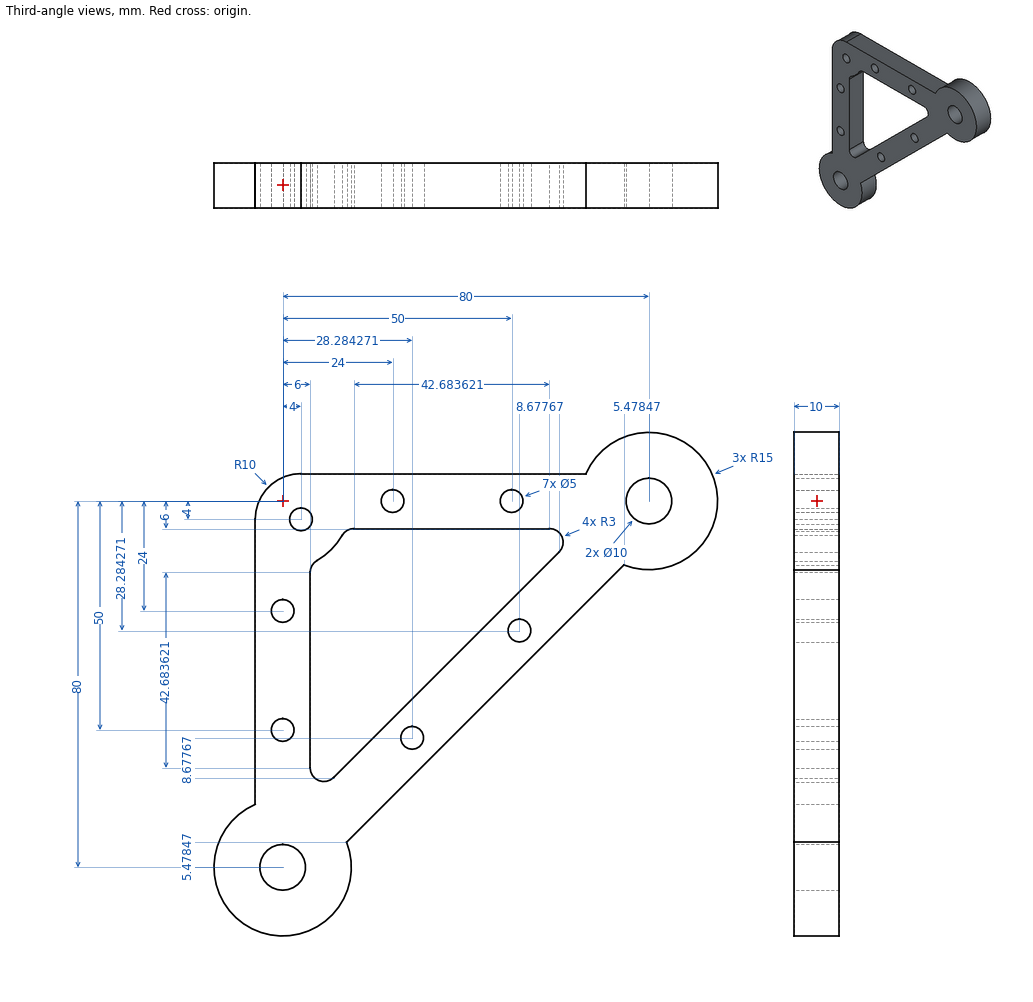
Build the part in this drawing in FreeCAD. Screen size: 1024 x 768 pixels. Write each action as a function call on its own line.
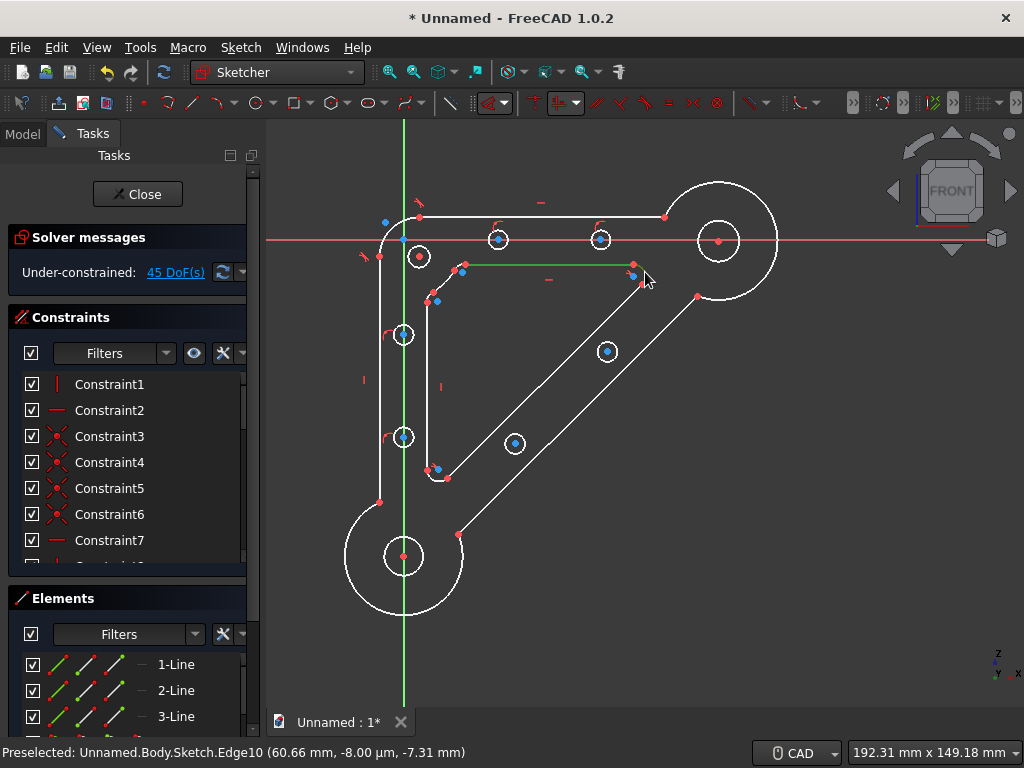
key(t)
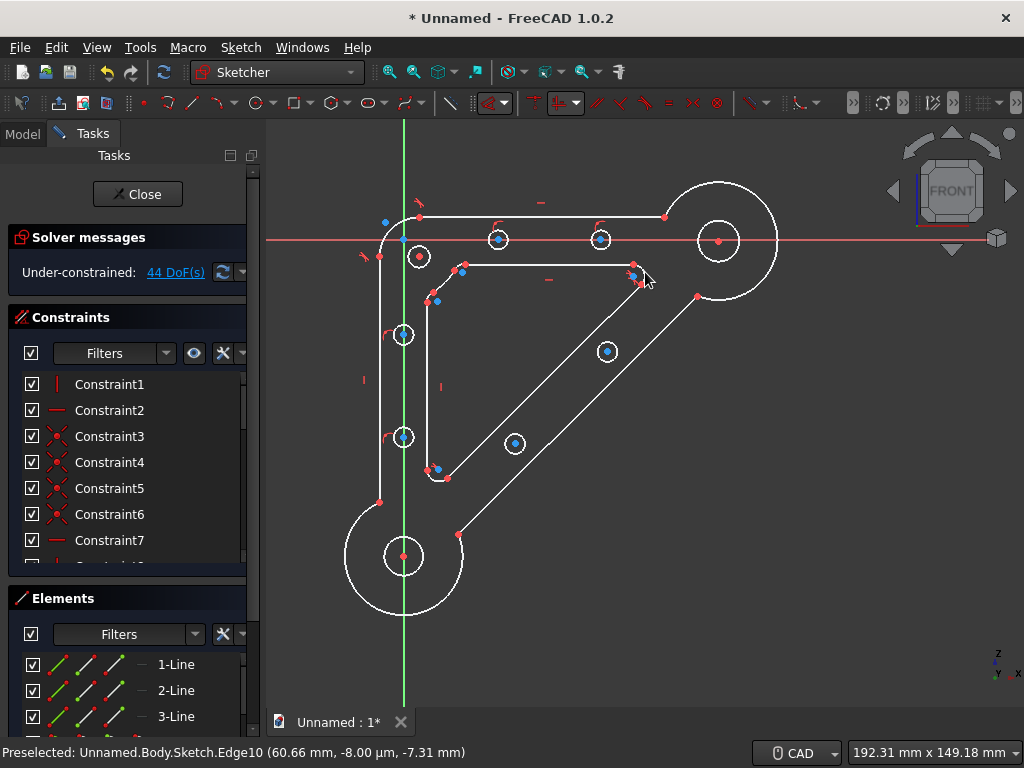
click(583, 265)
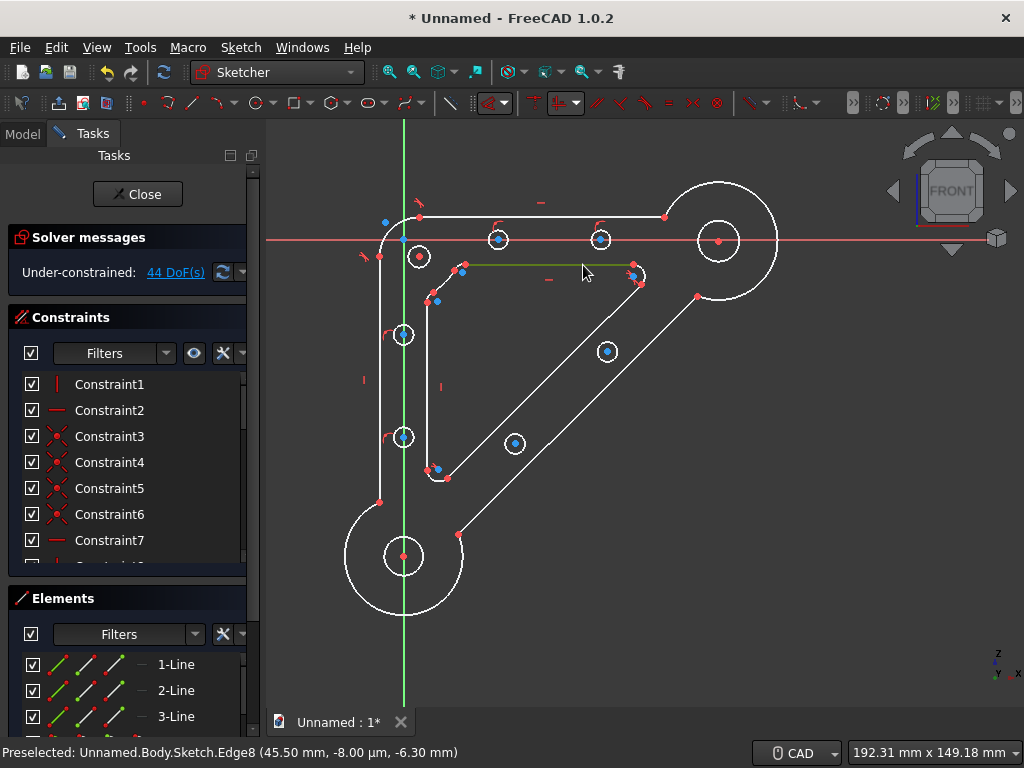
scroll(459, 265, up, 4)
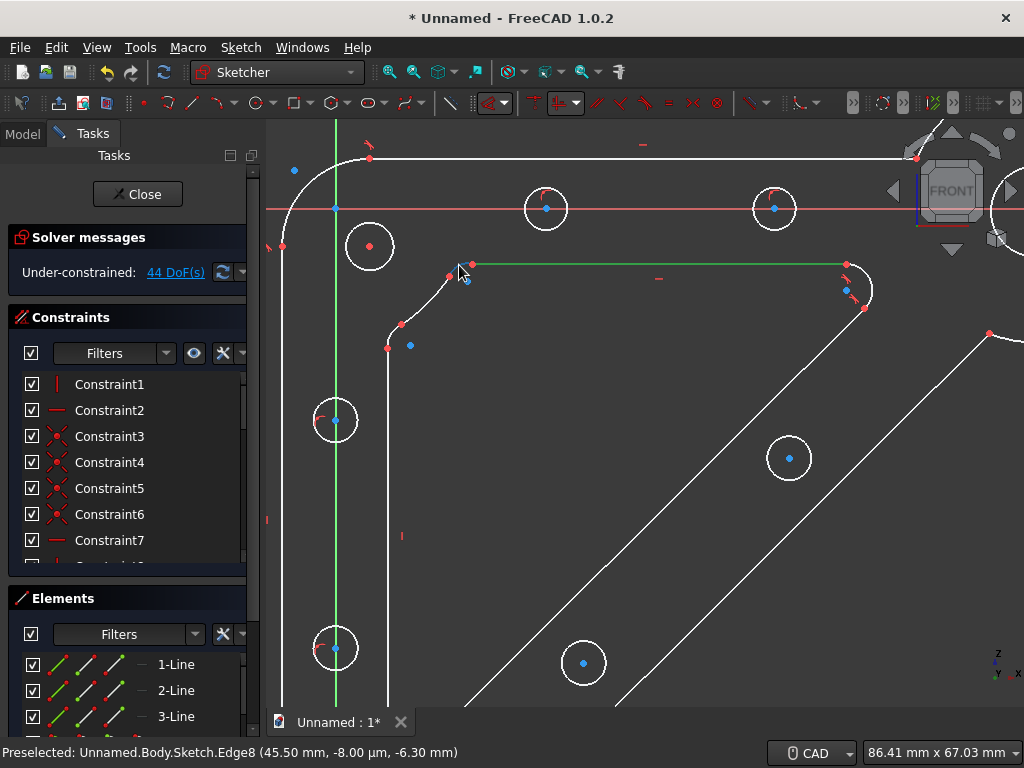
click(458, 266)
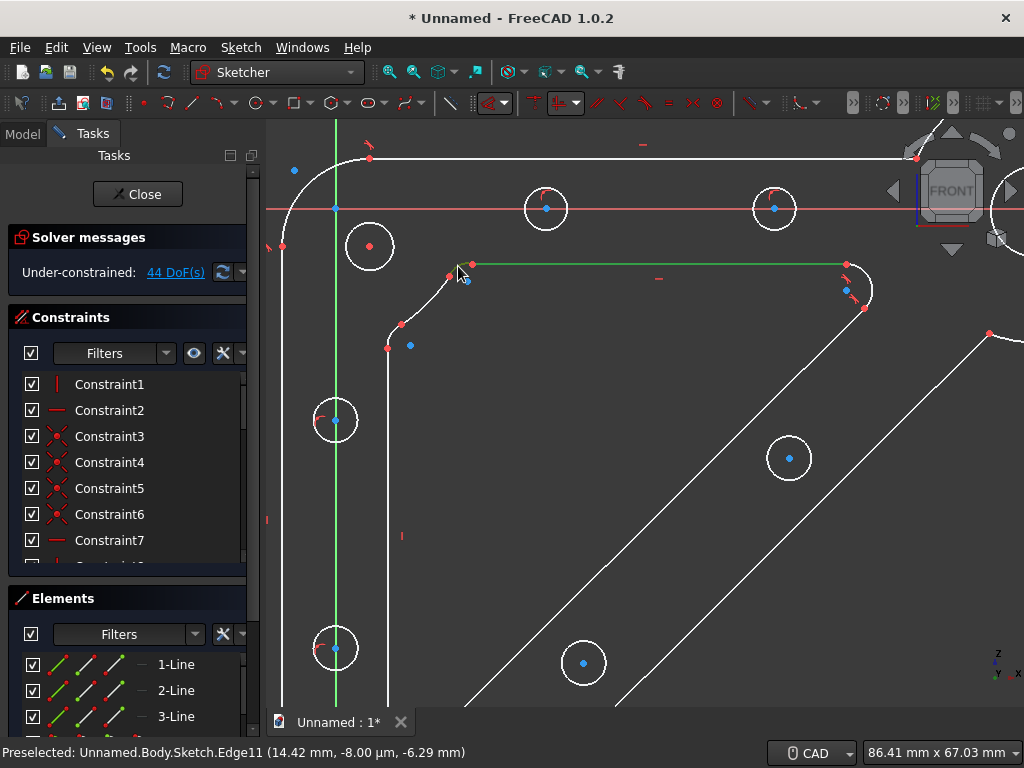
click(646, 104)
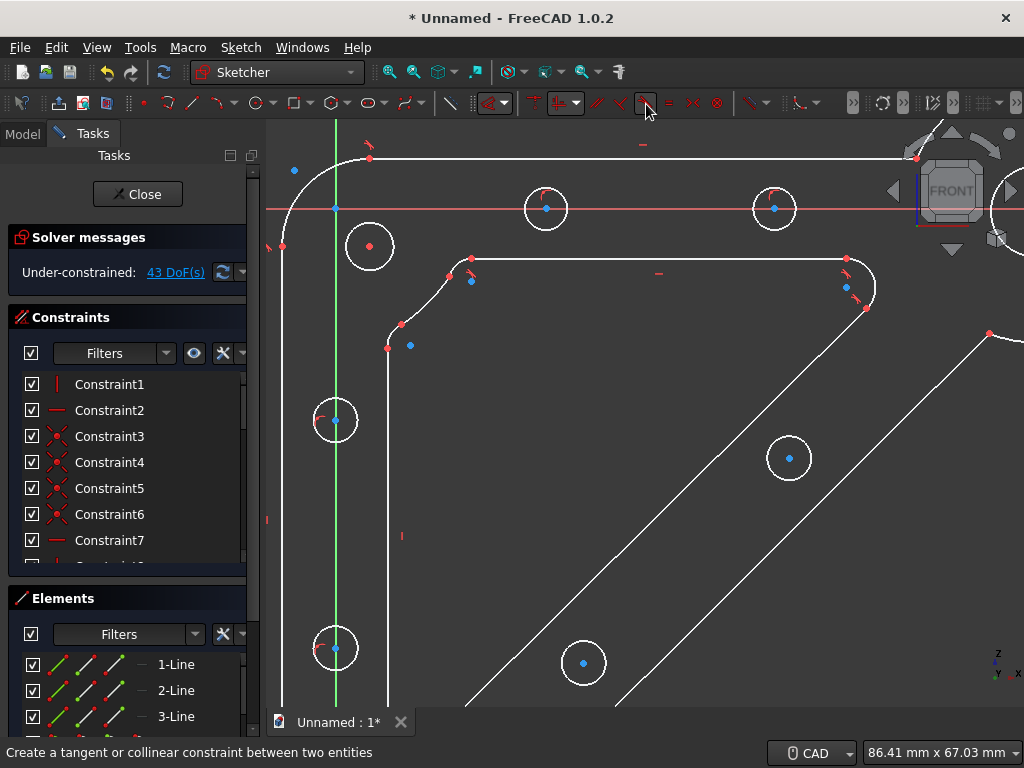
click(388, 461)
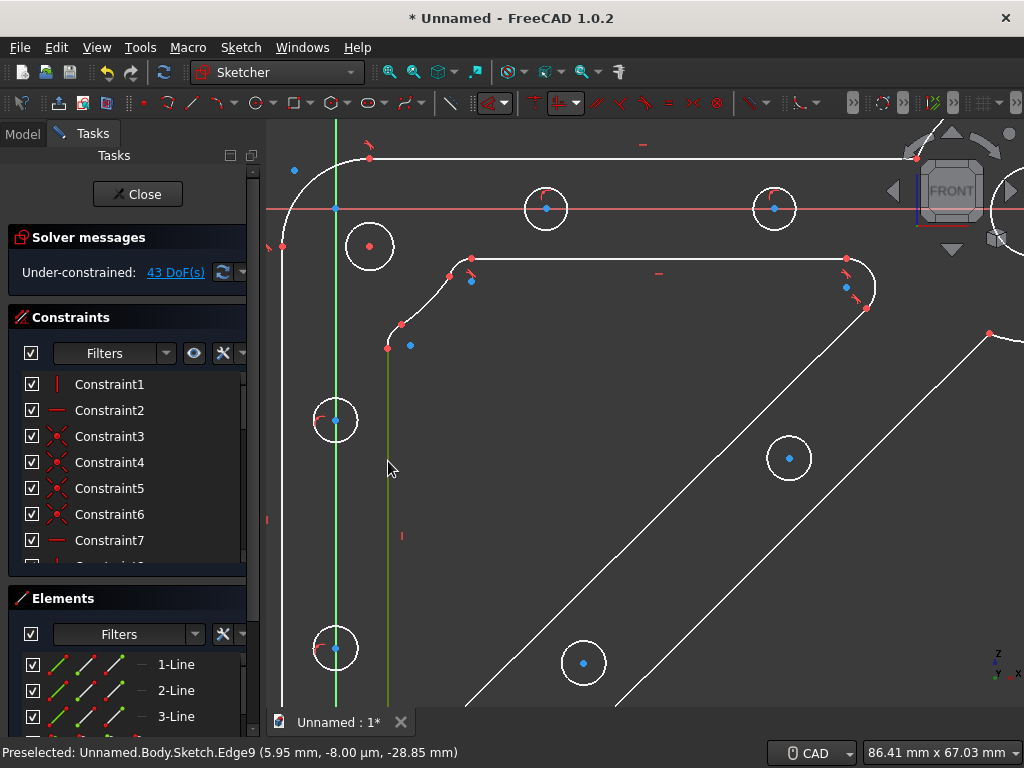
click(391, 334)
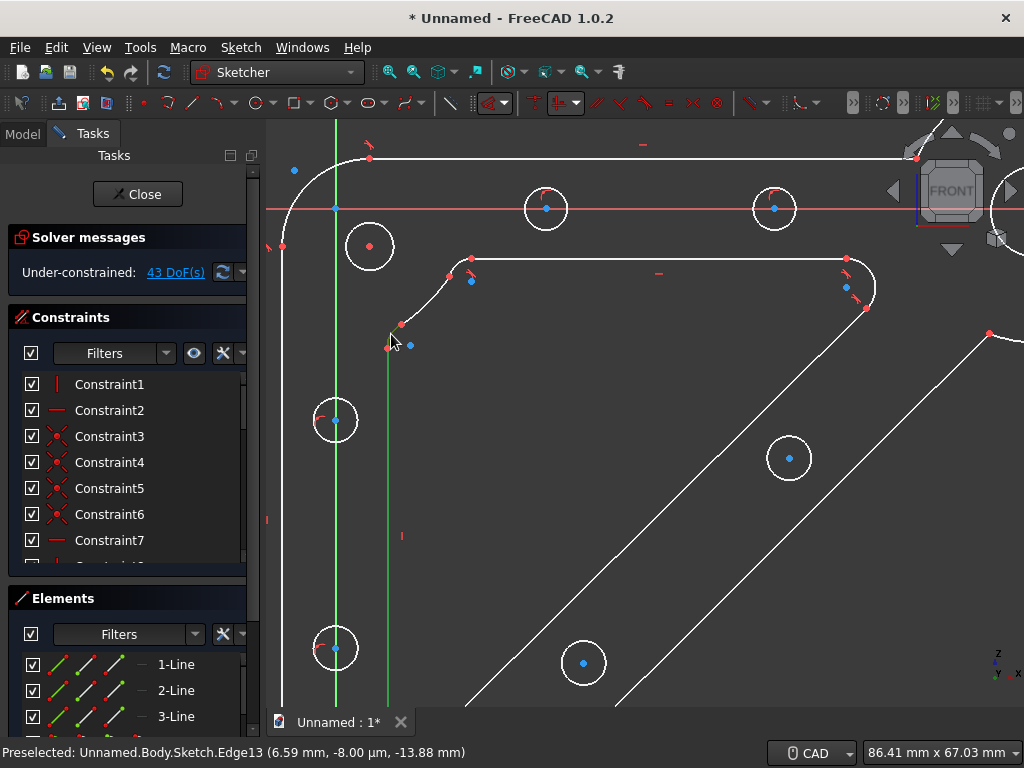
click(646, 104)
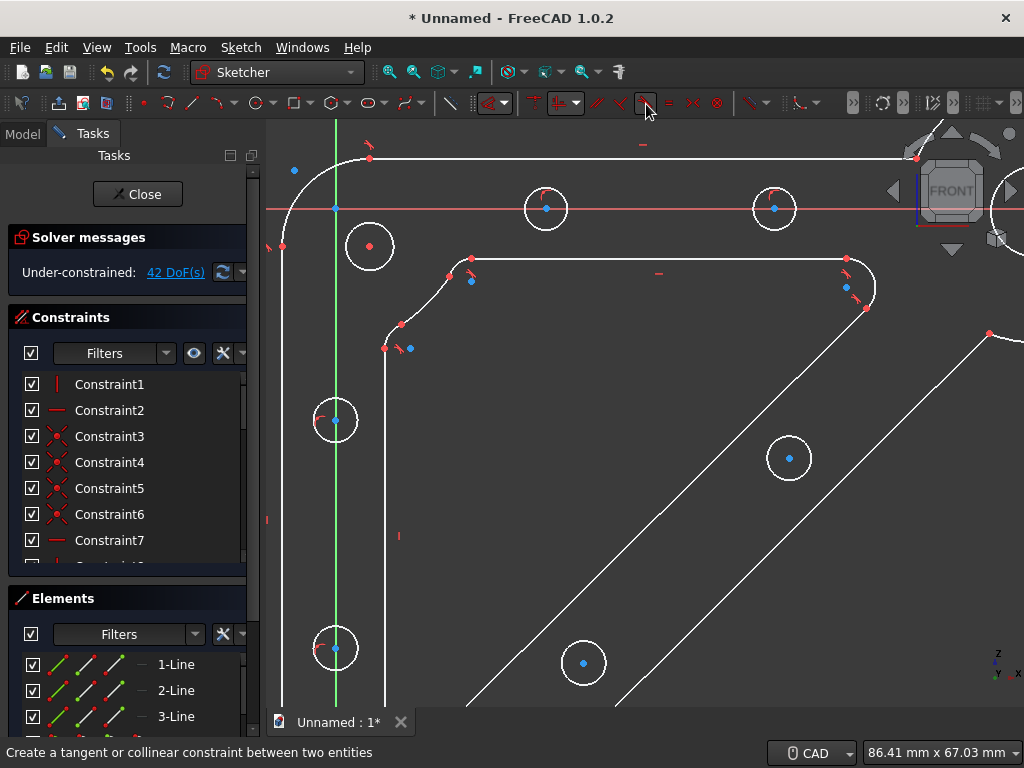
click(385, 461)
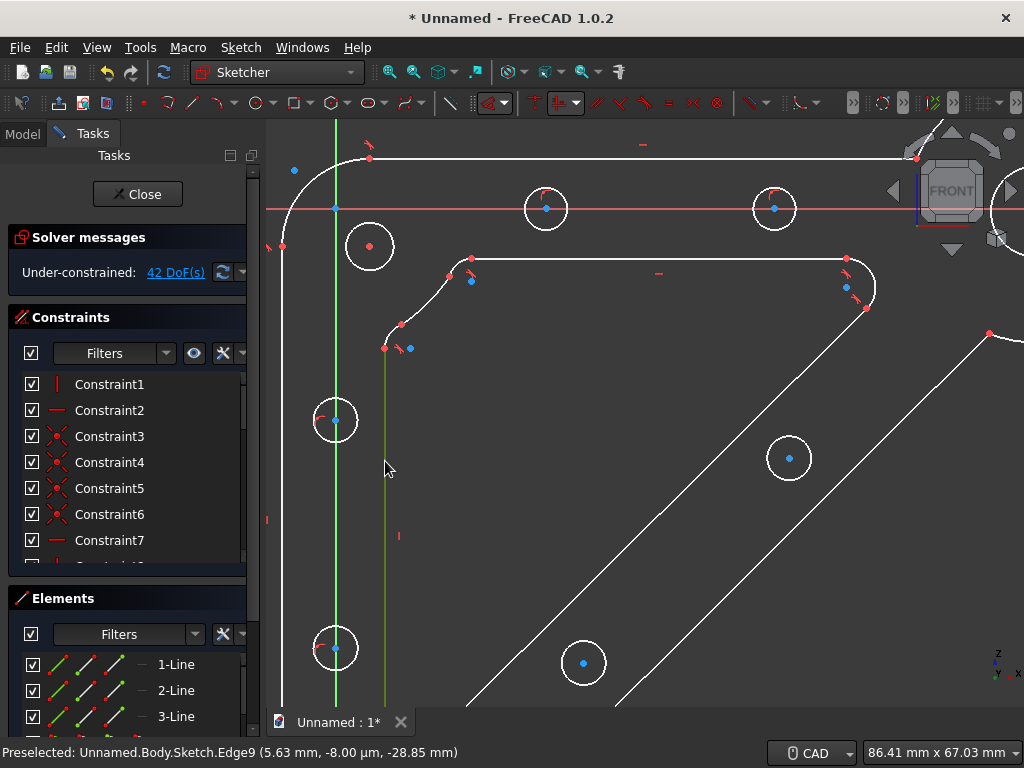
scroll(459, 265, down, 4)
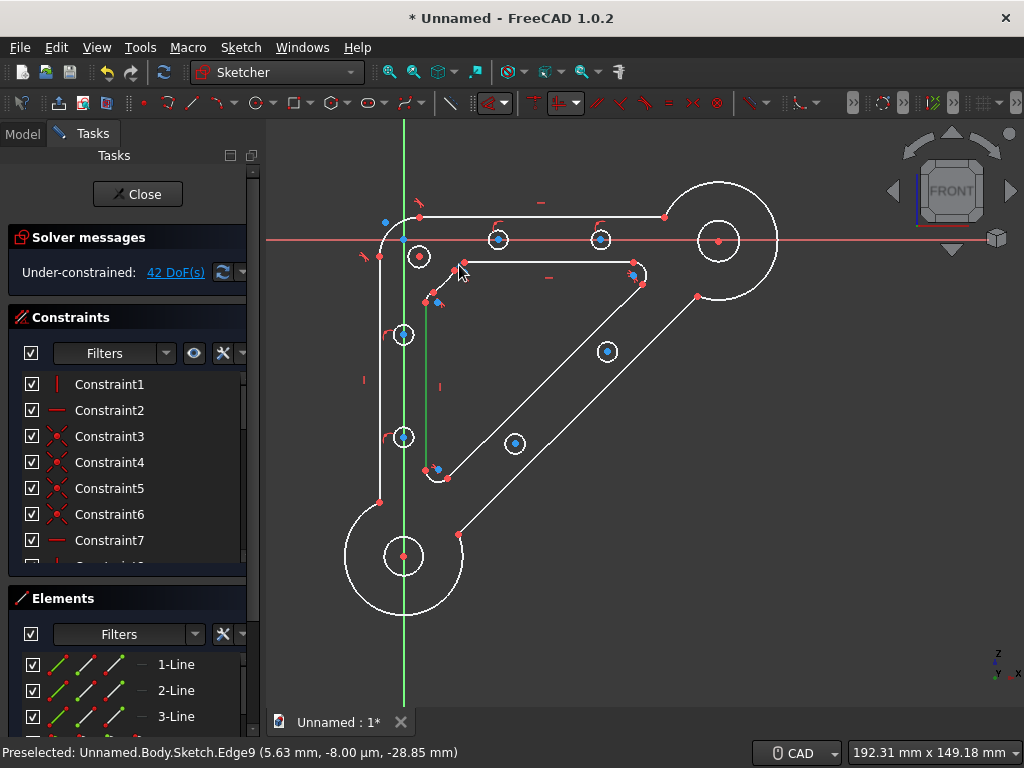
scroll(429, 478, up, 3)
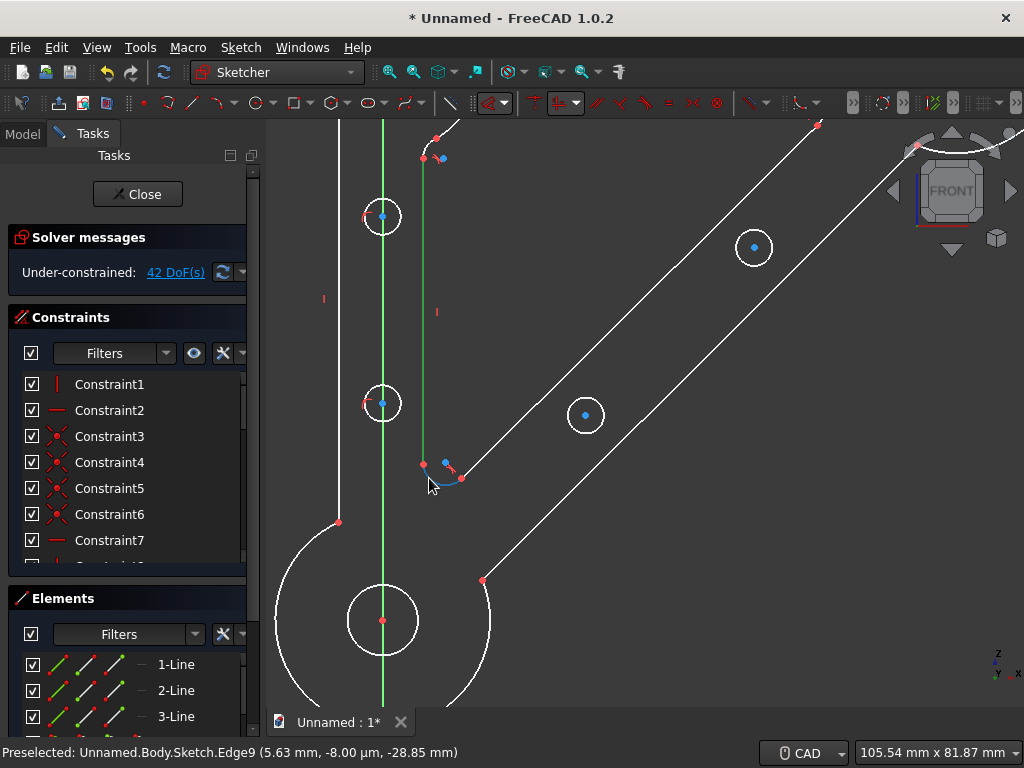
click(429, 478)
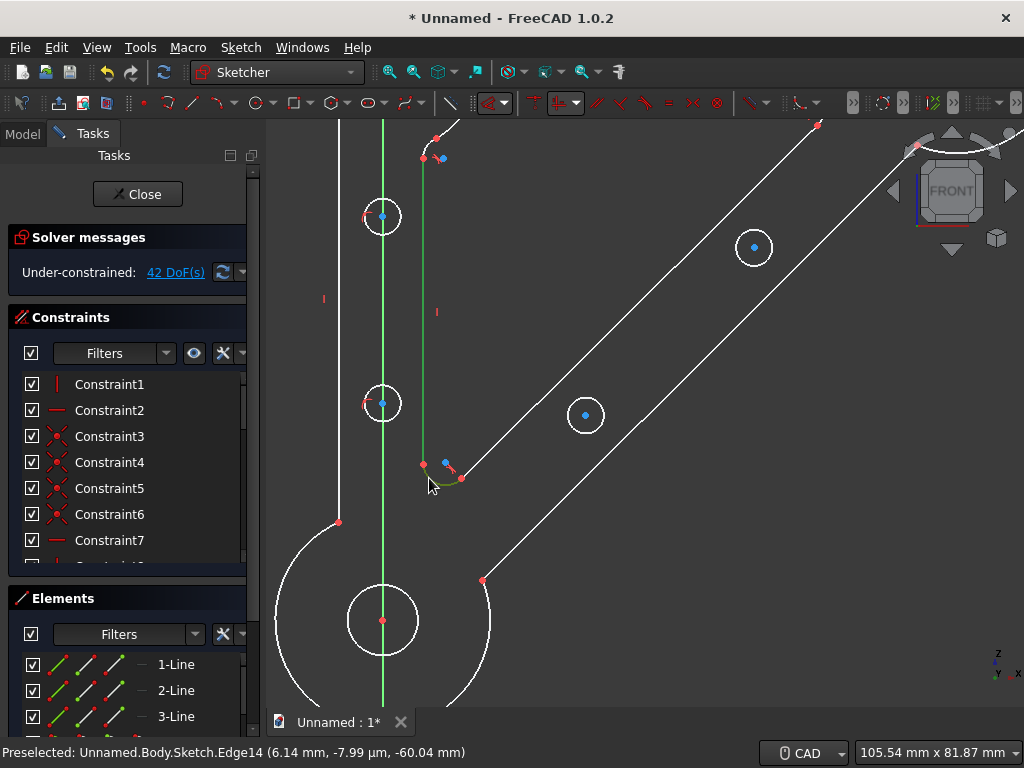
click(646, 104)